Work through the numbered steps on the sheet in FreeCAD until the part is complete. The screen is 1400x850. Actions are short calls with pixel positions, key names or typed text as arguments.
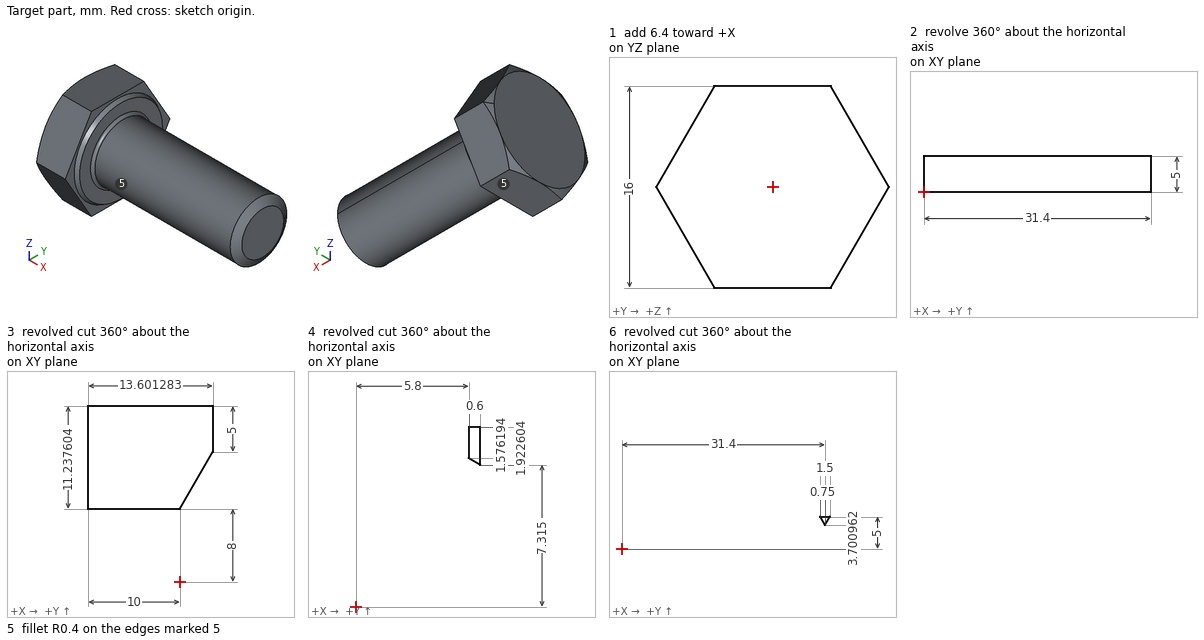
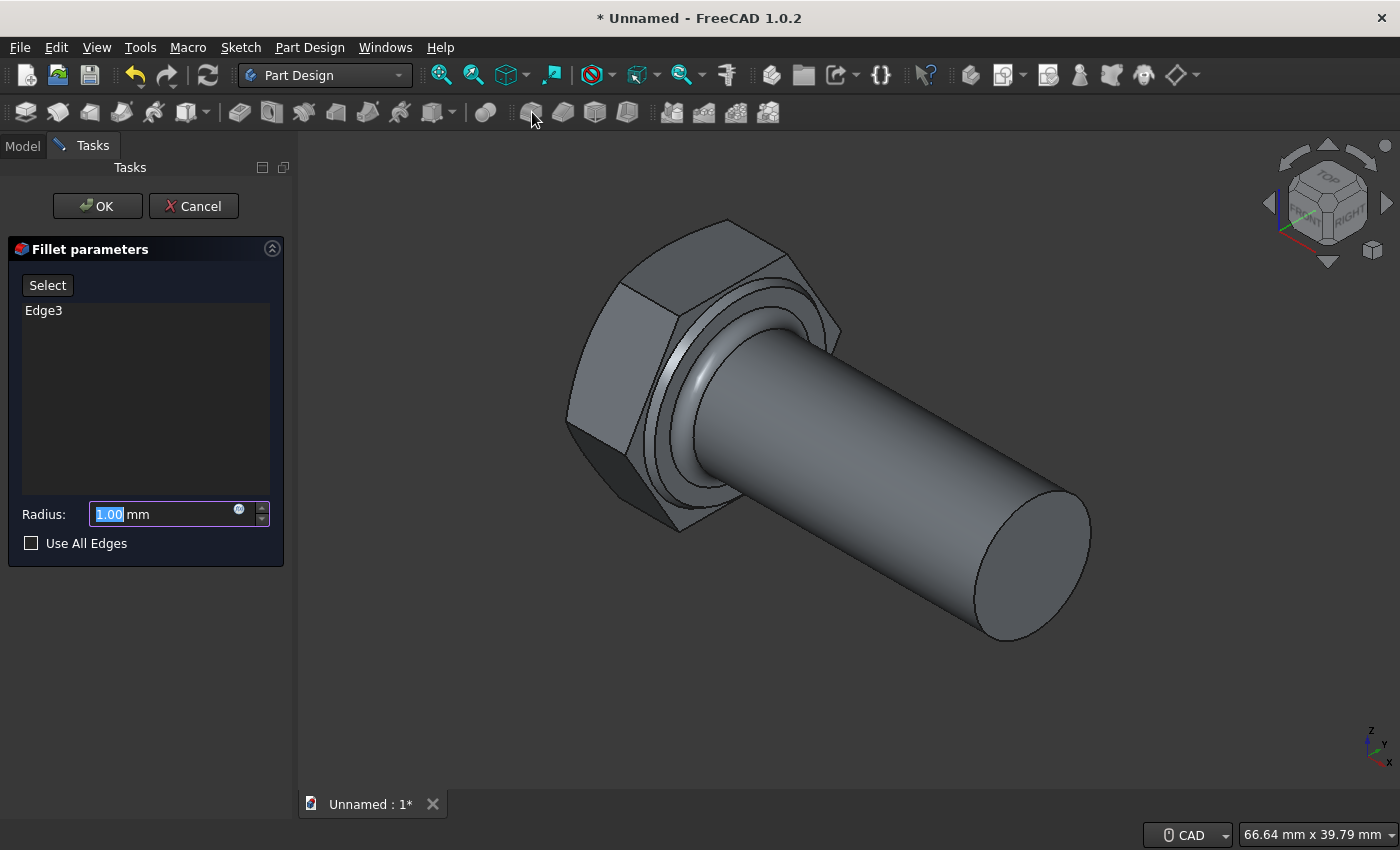
text(0.4)
key(Tab)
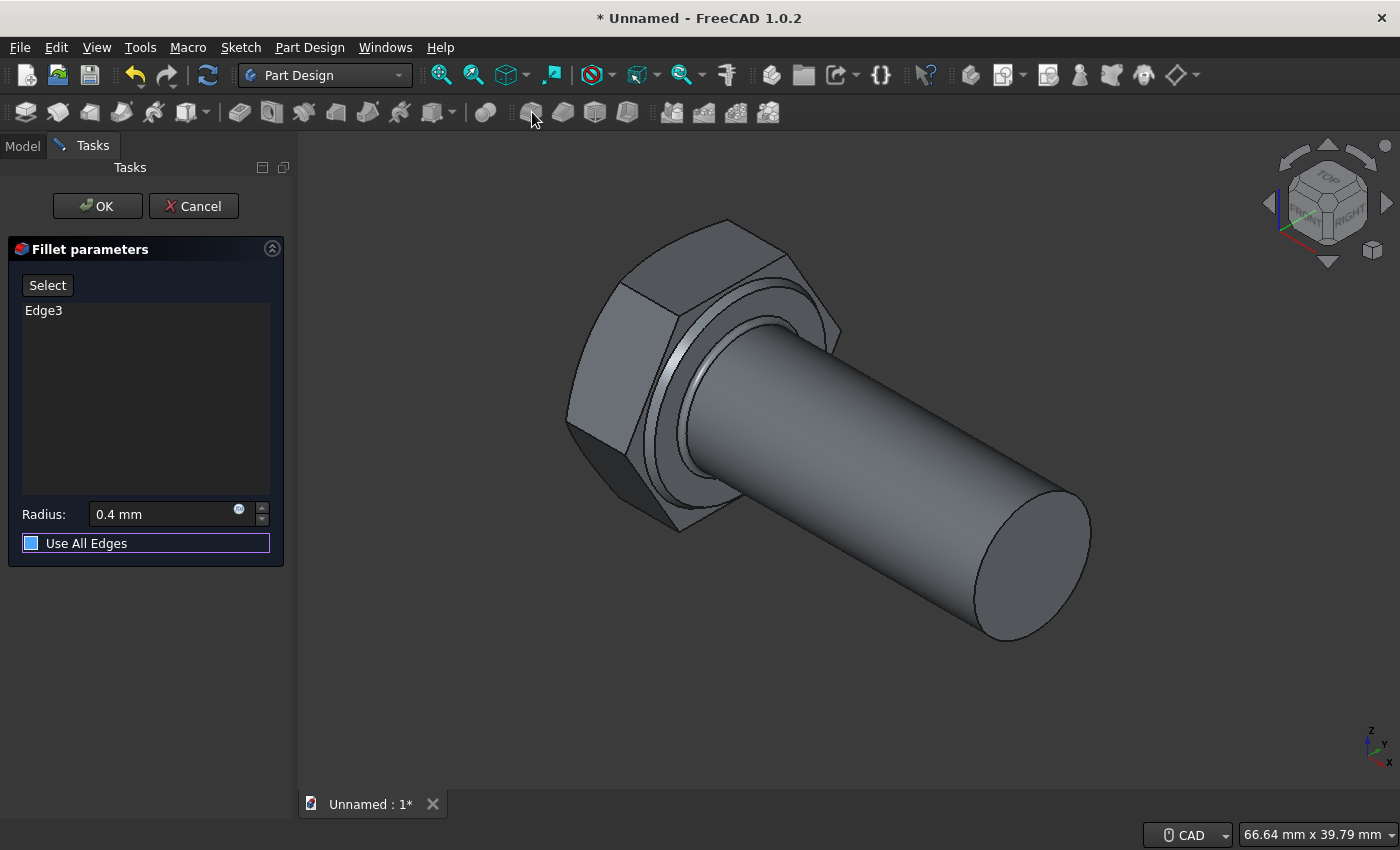
click(98, 206)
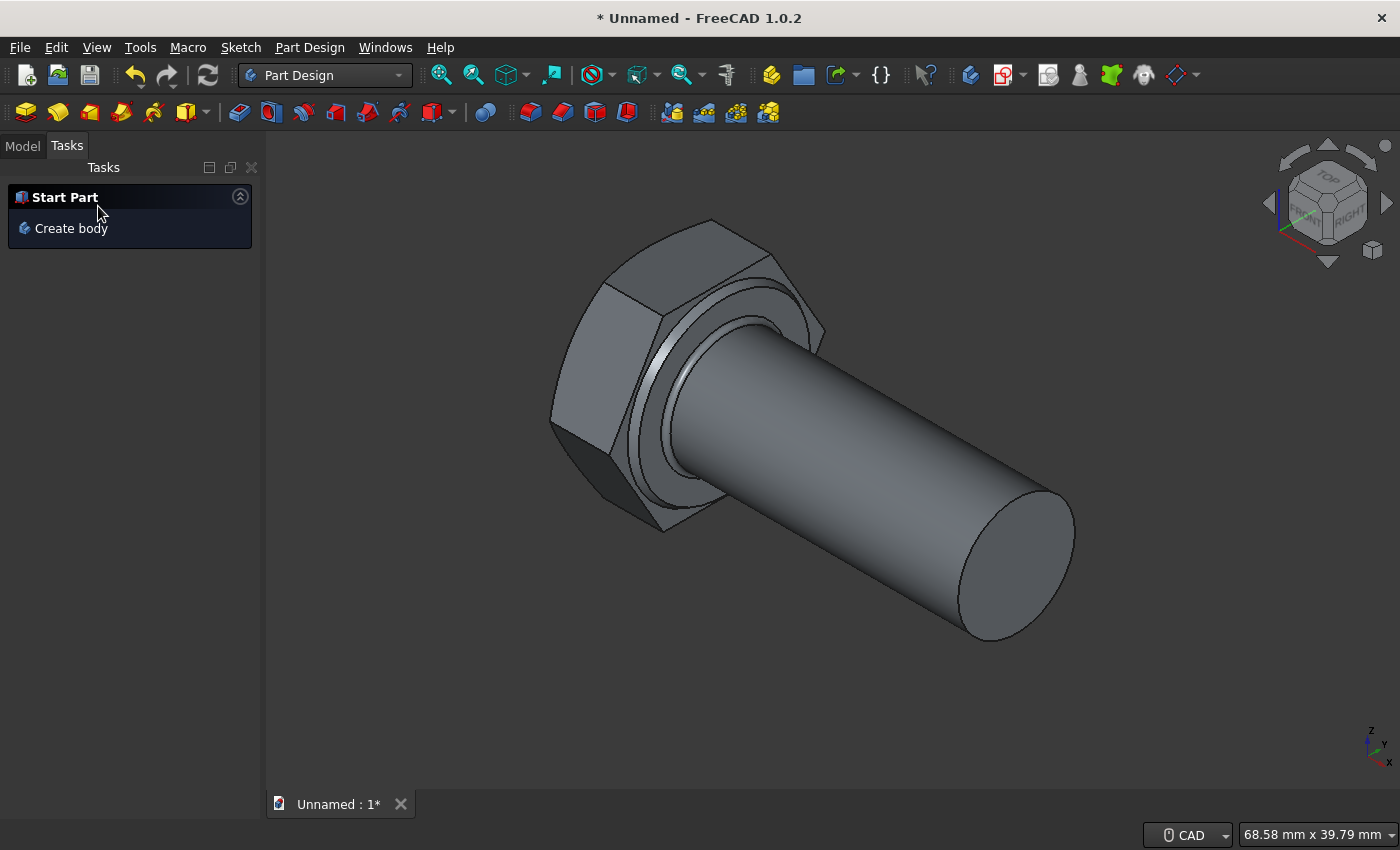
click(1004, 76)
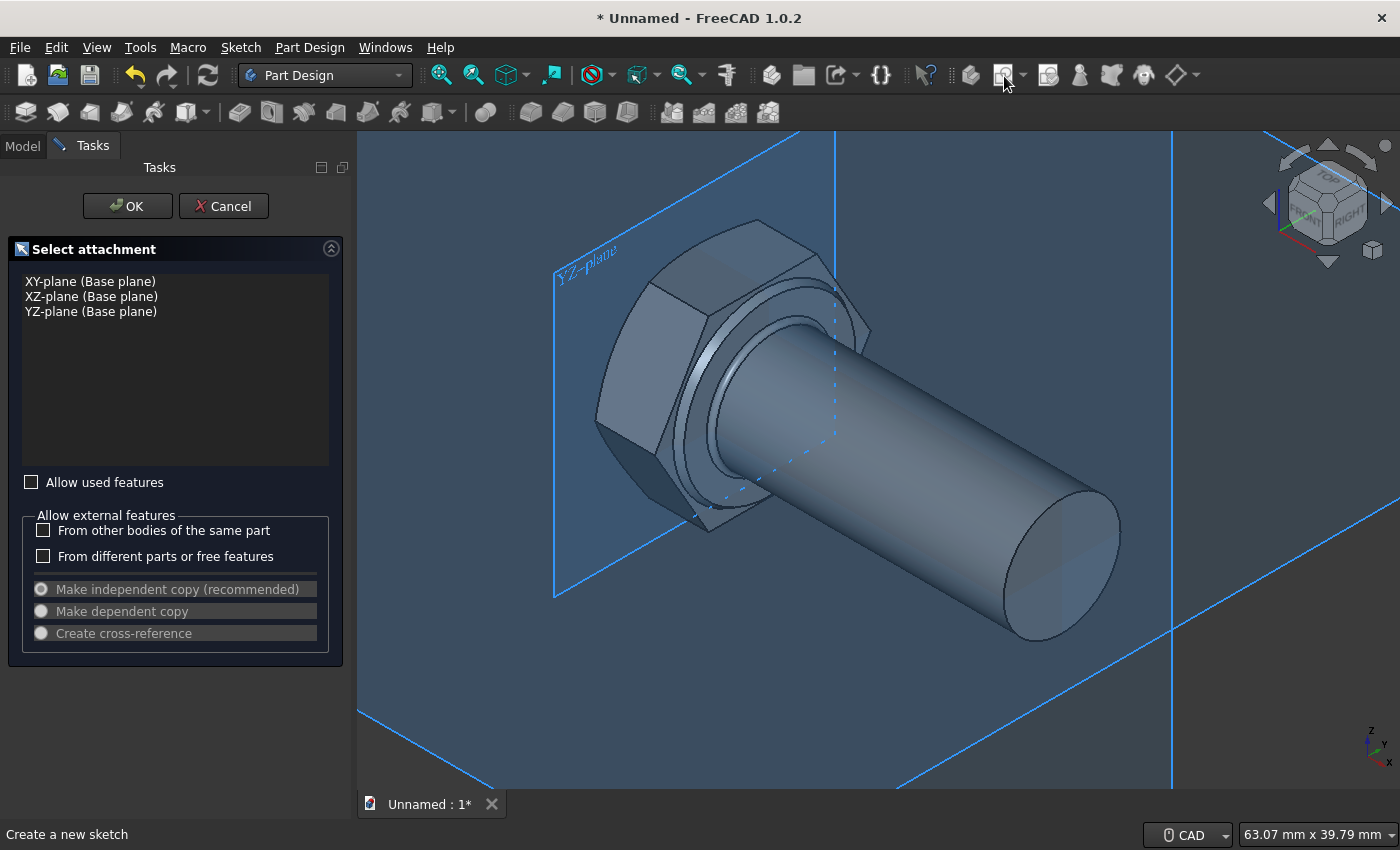
click(82, 282)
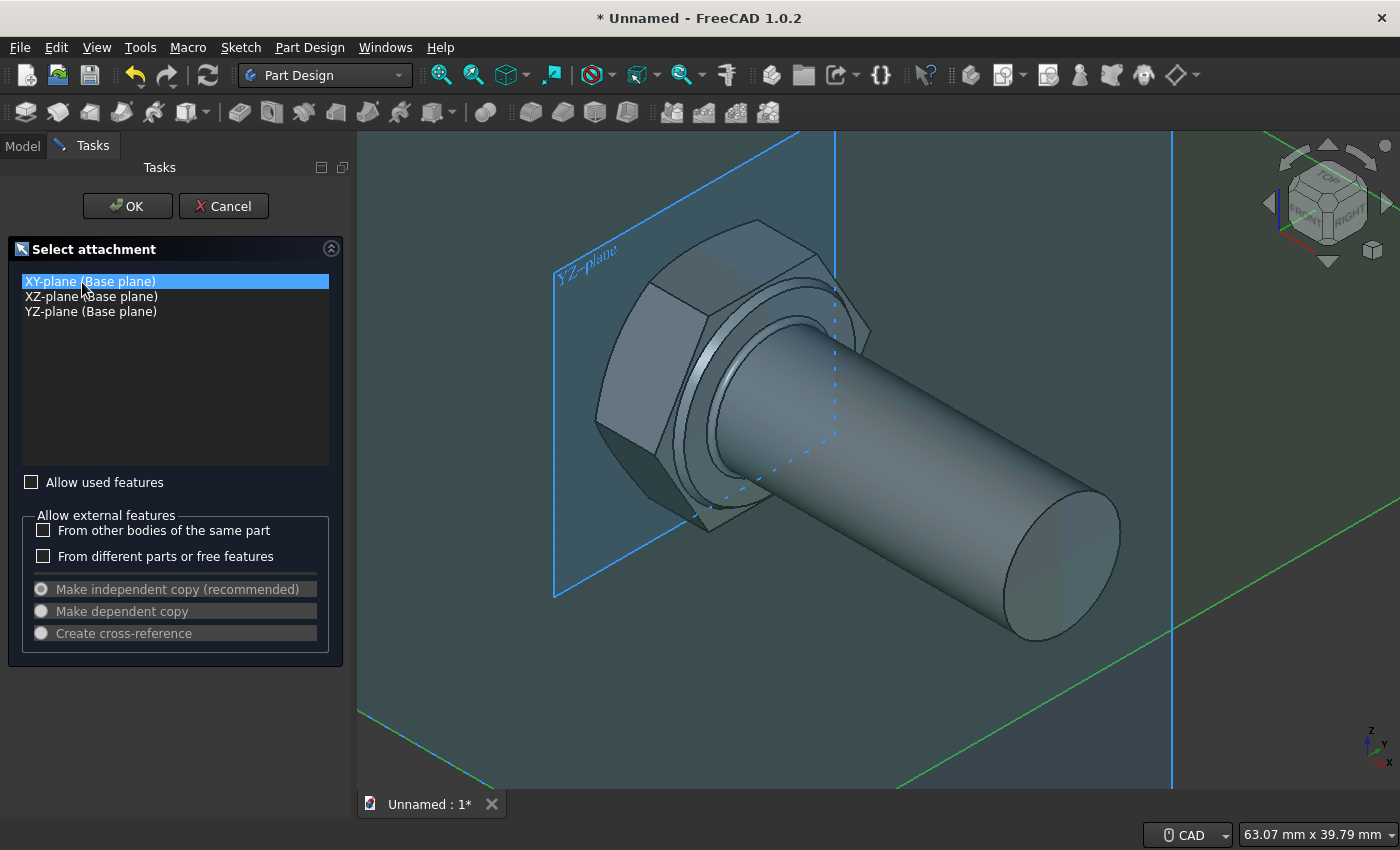
click(128, 206)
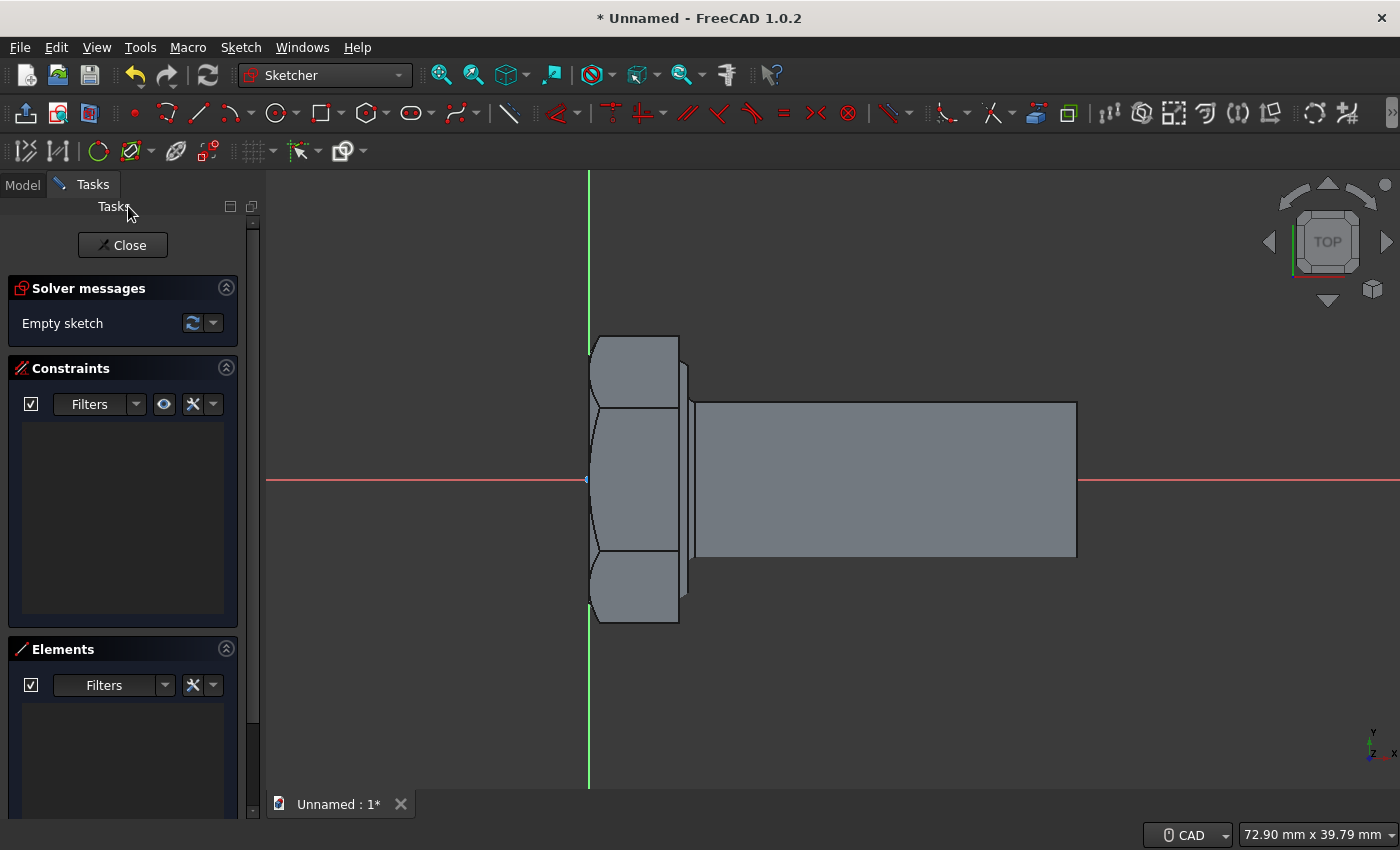
click(90, 114)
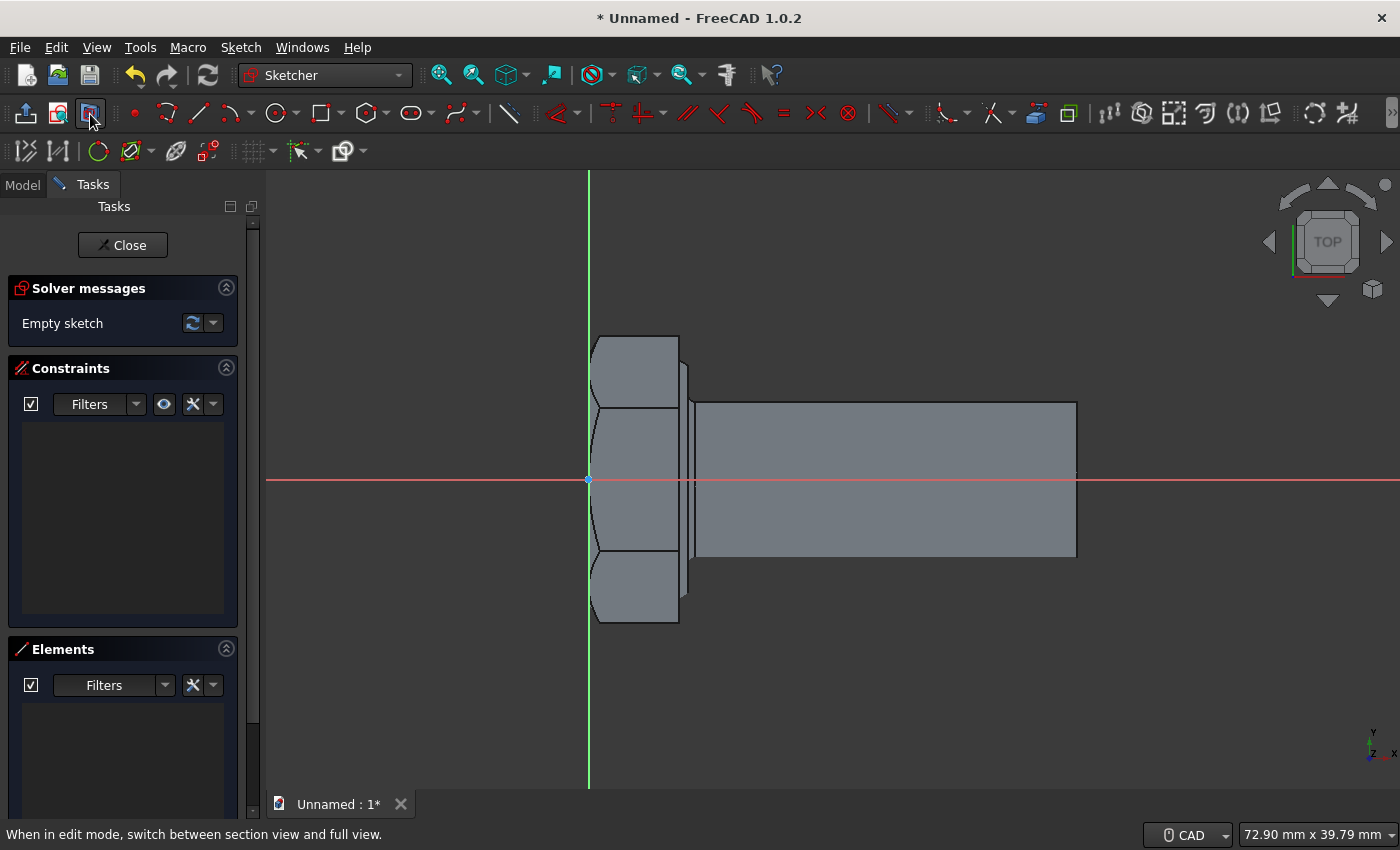
scroll(1094, 408, up, 15)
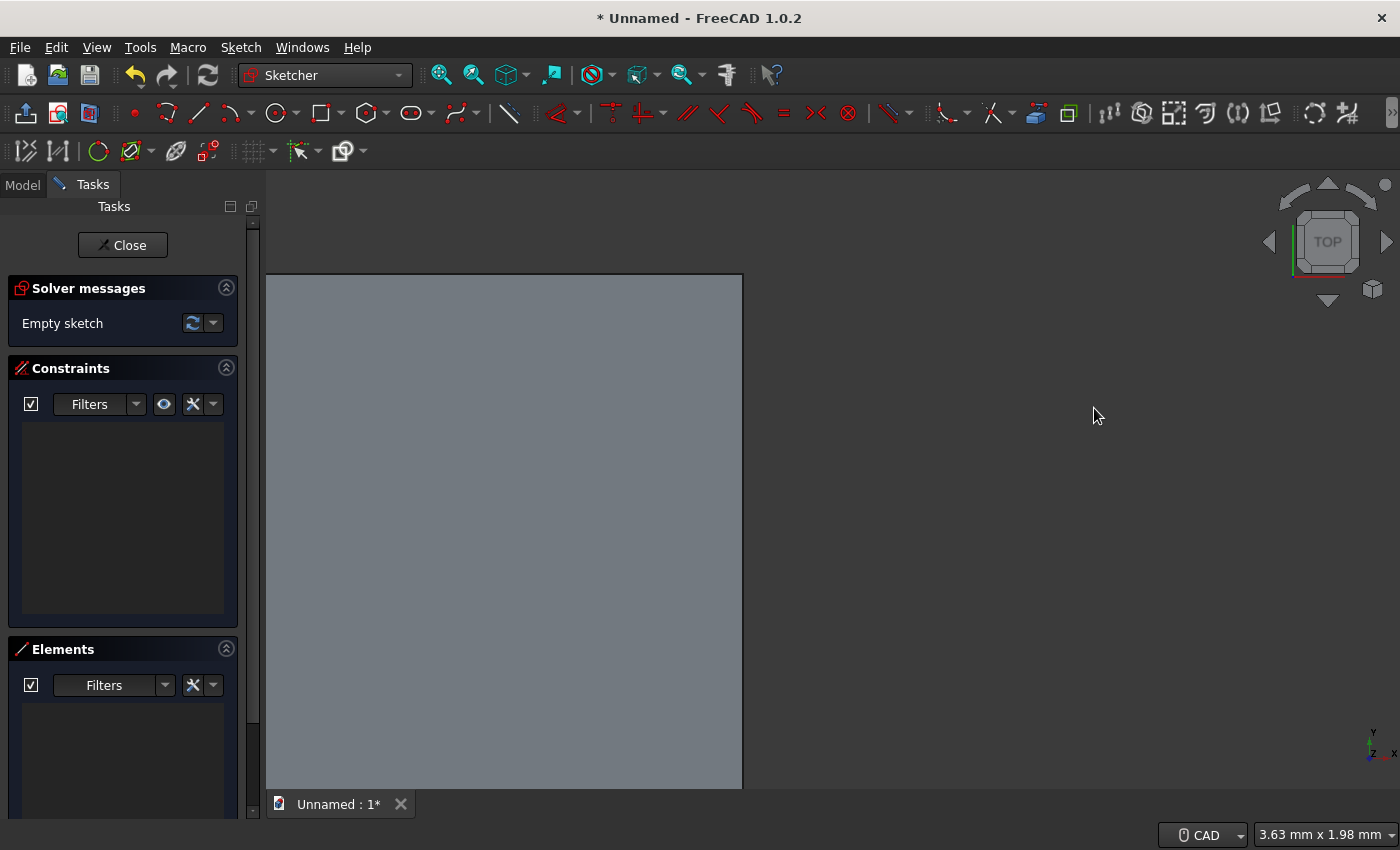
click(168, 114)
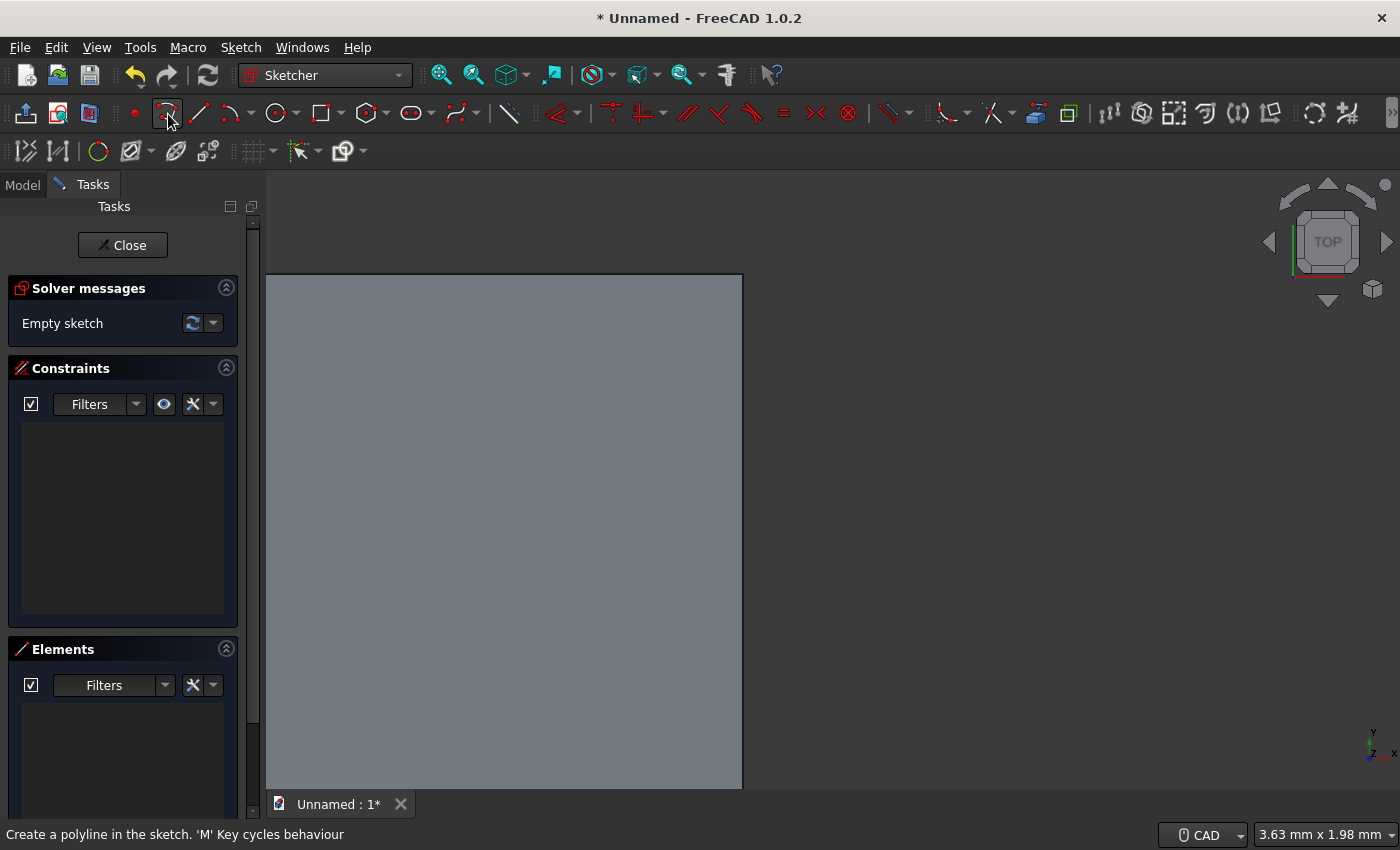
click(509, 274)
click(743, 680)
click(978, 274)
click(509, 275)
key(Escape)
key(Escape)